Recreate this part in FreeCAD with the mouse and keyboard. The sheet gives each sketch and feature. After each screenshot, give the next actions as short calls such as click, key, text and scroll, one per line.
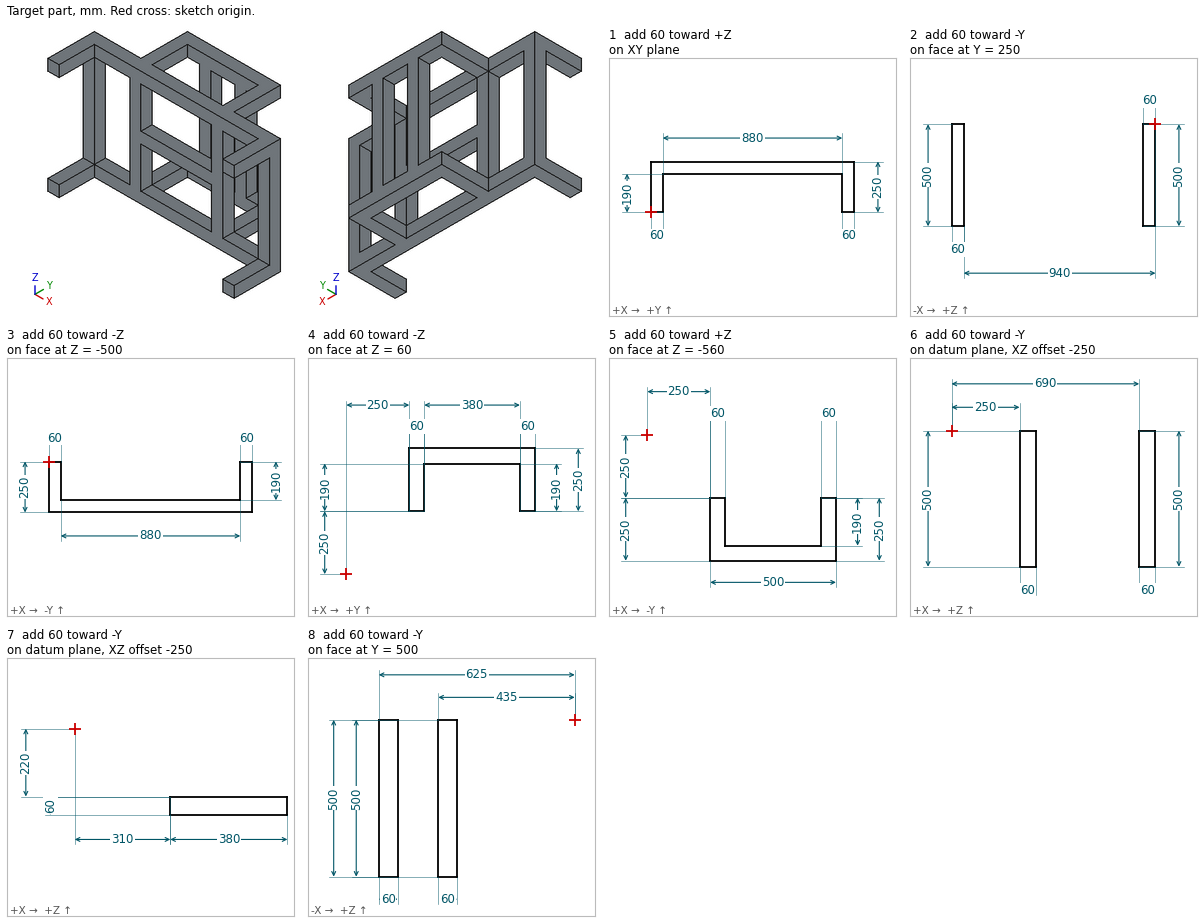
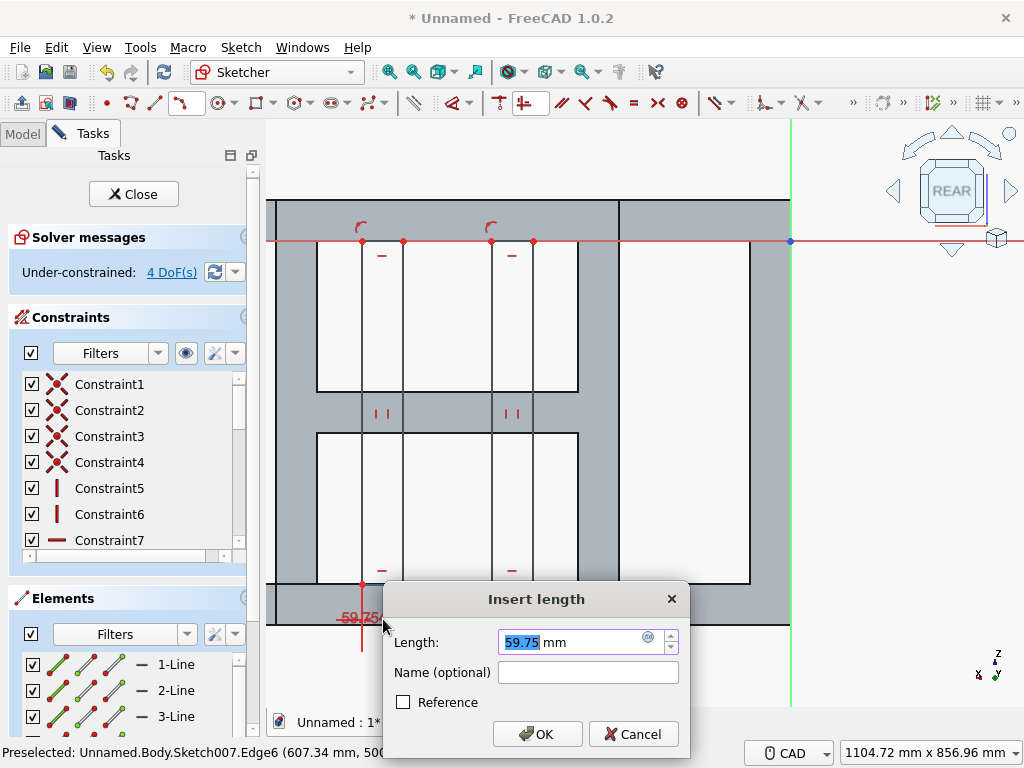
text(60)
key(Return)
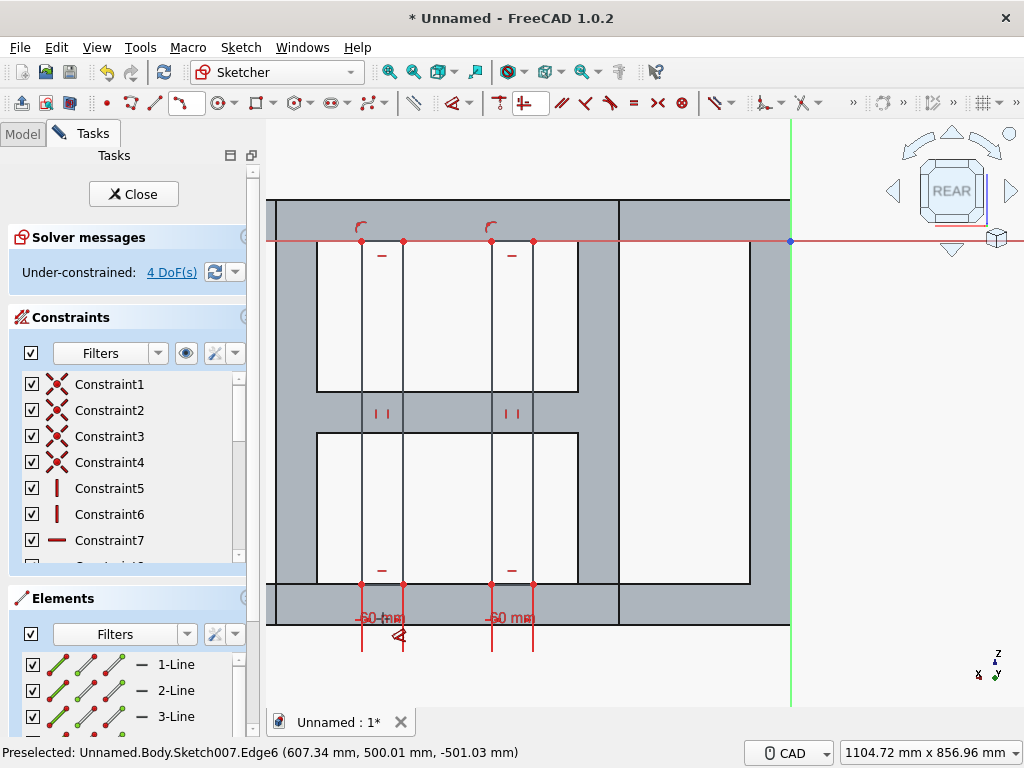
click(492, 344)
click(458, 413)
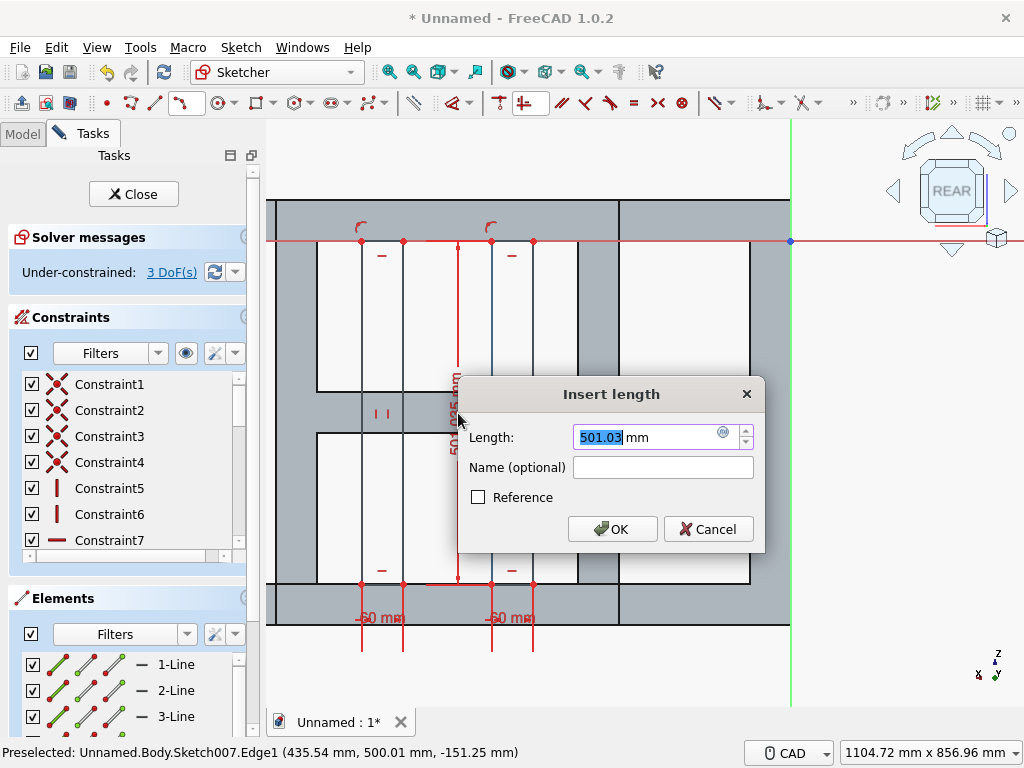
text(500)
key(Return)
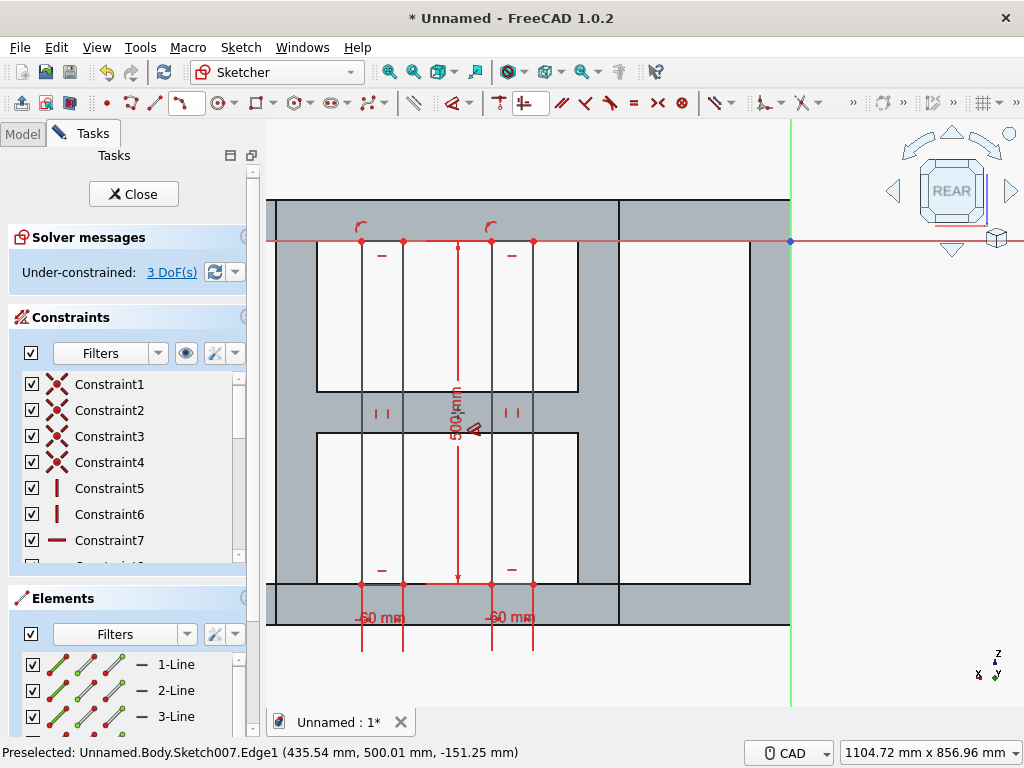
click(362, 344)
click(328, 413)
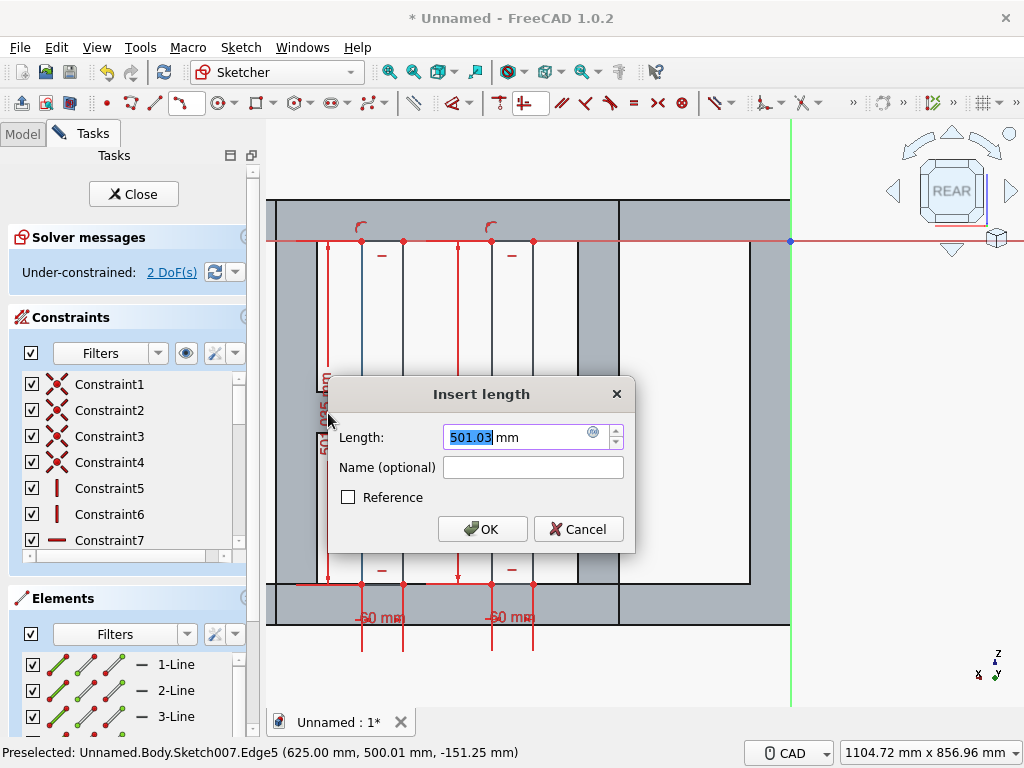
text(500)
key(Return)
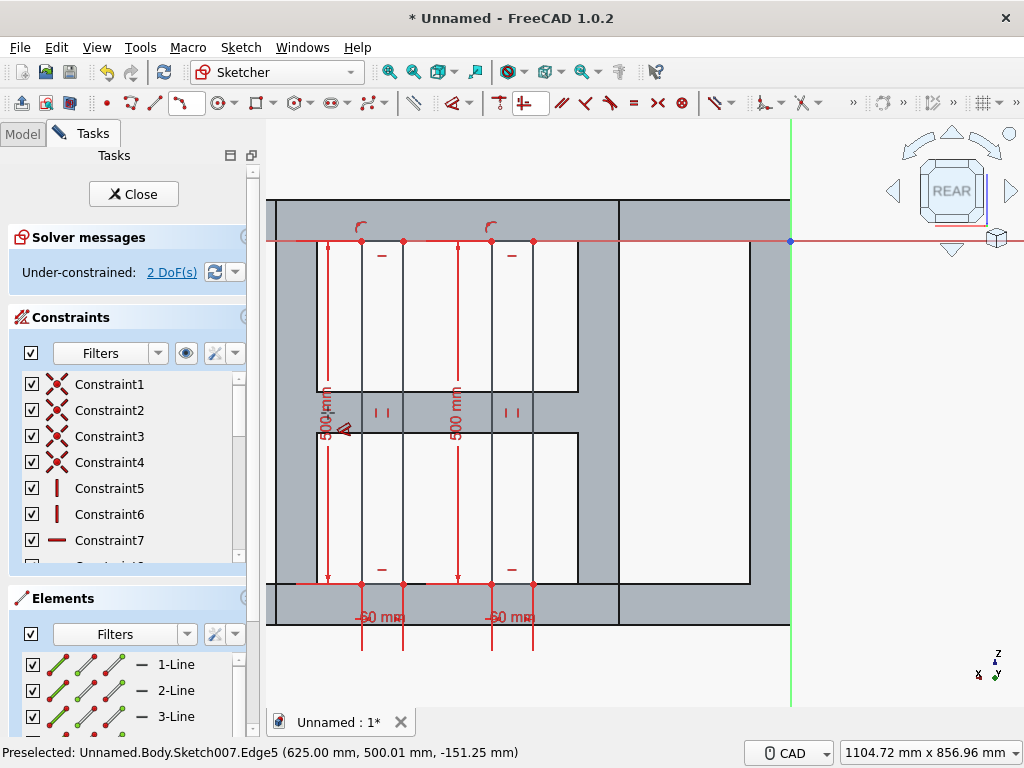
click(492, 241)
click(641, 207)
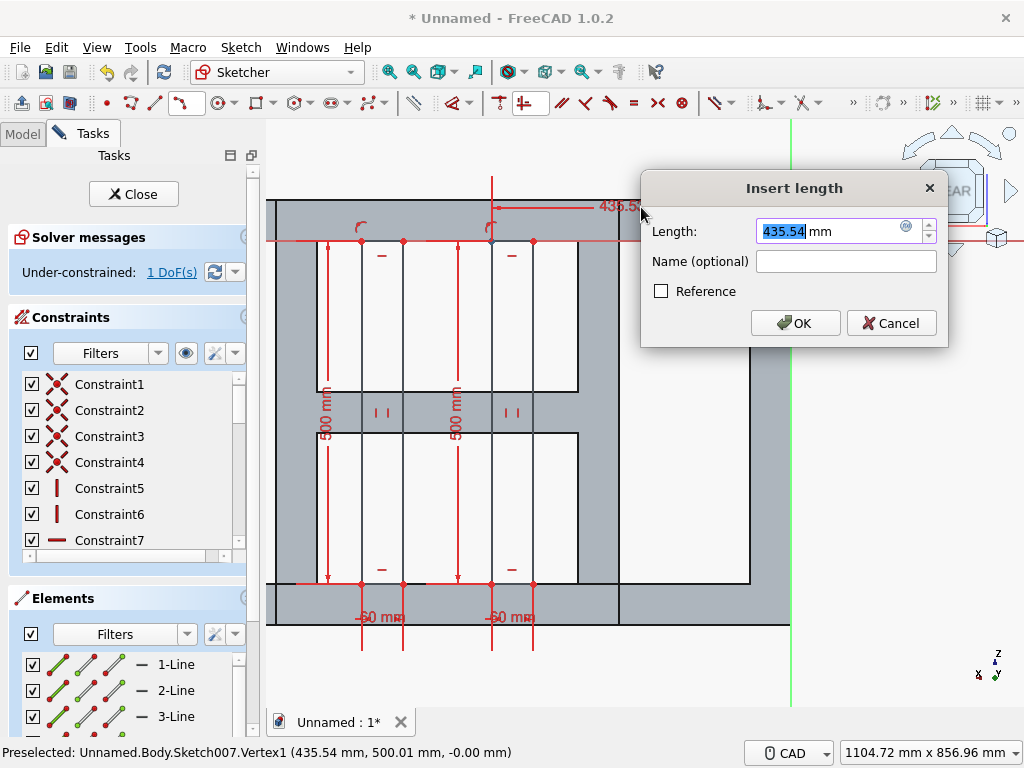
text(435)
key(Return)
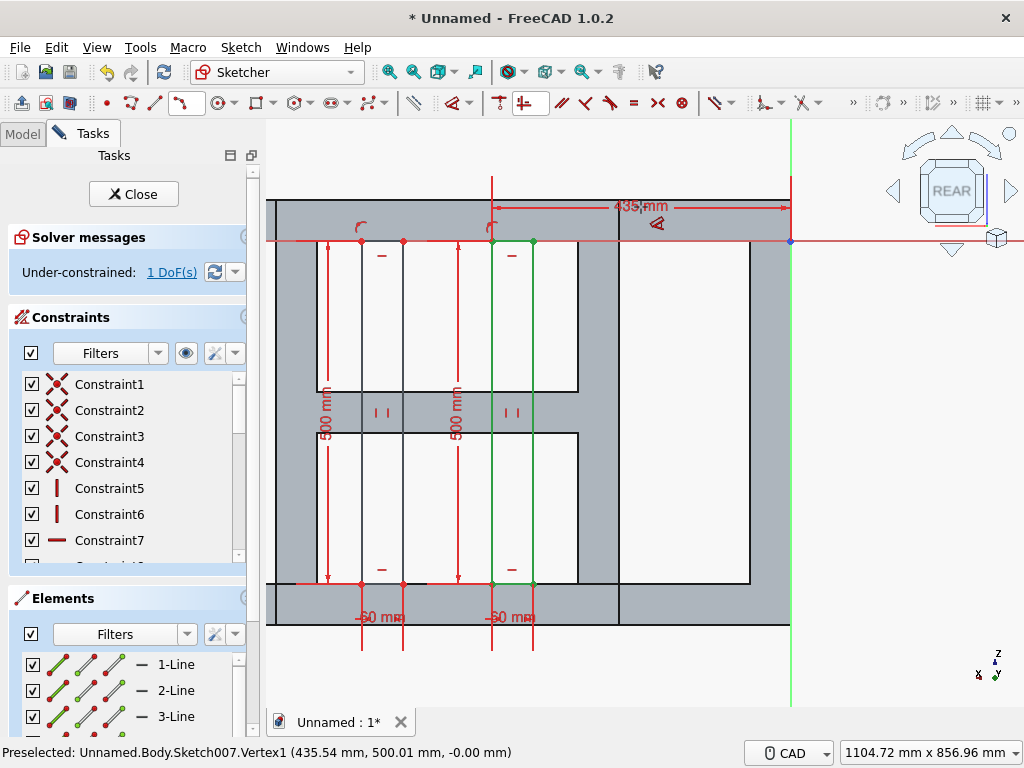
click(362, 241)
click(478, 207)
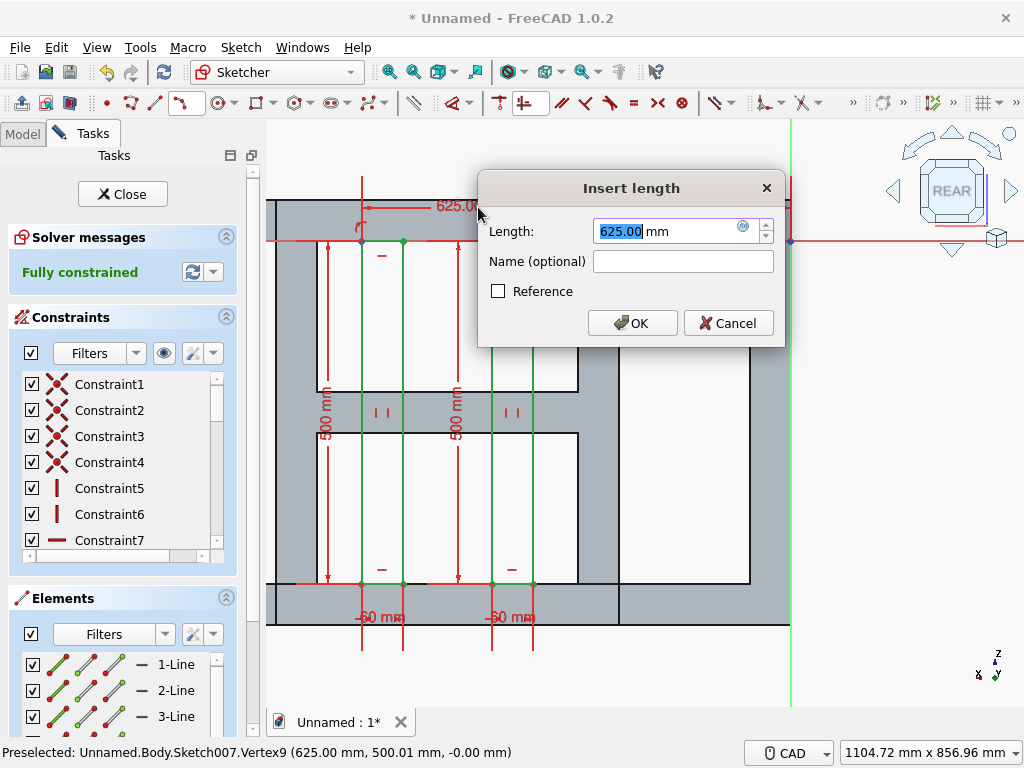
text(625)
key(Return)
key(Escape)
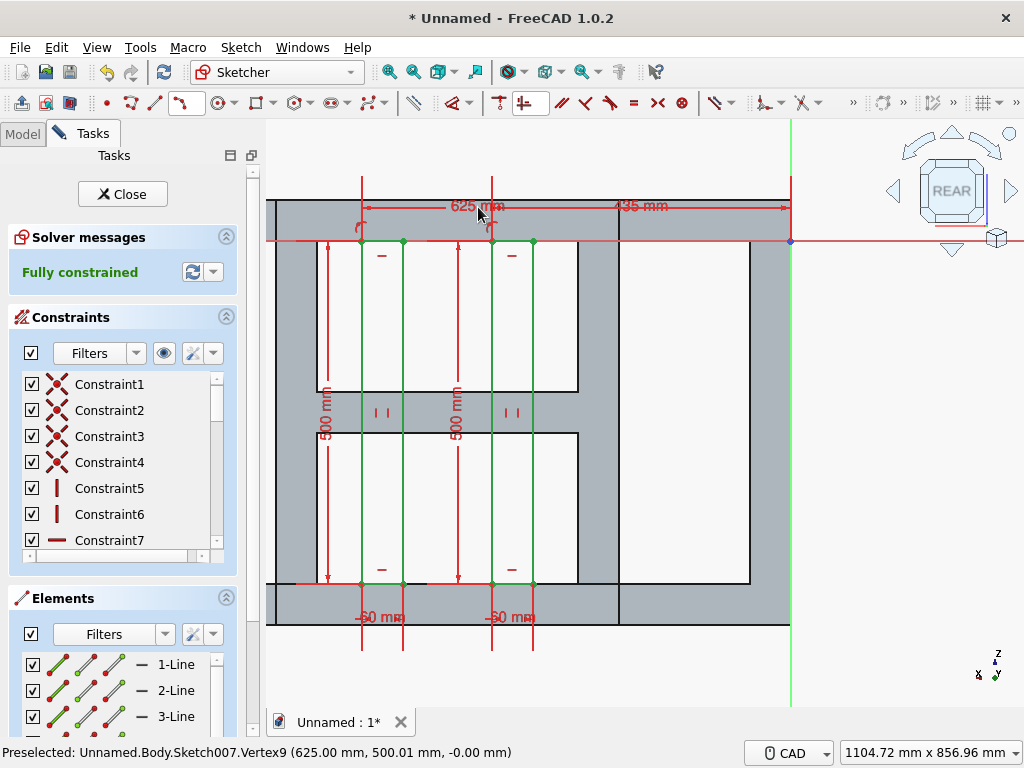
click(123, 194)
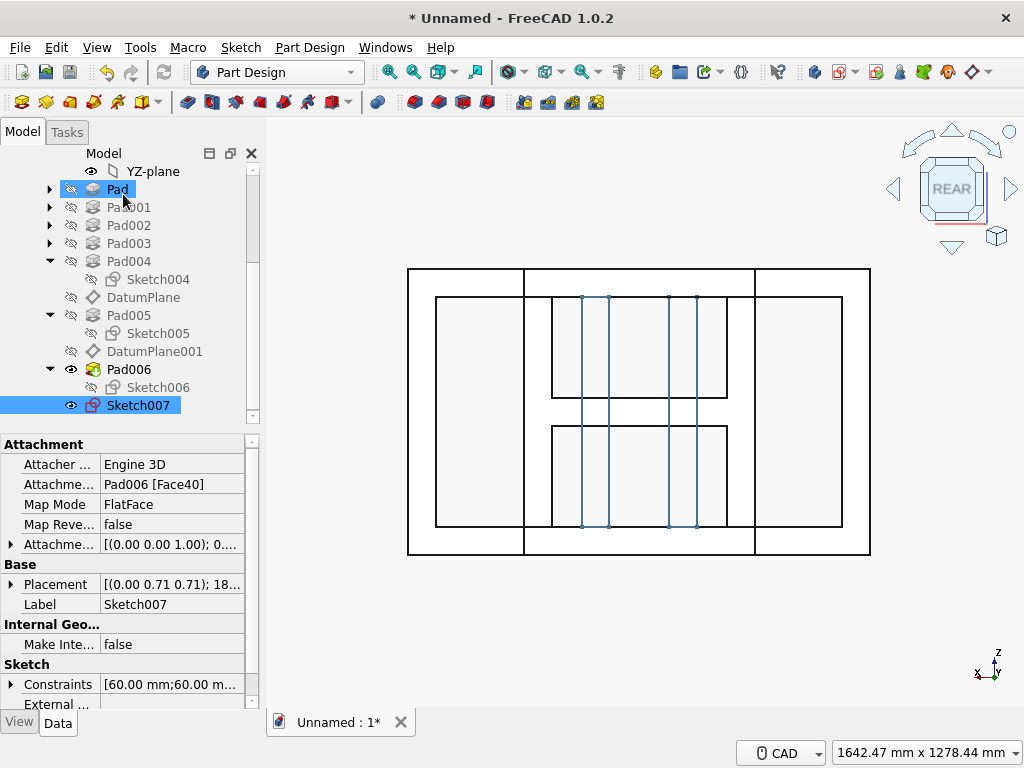
click(22, 102)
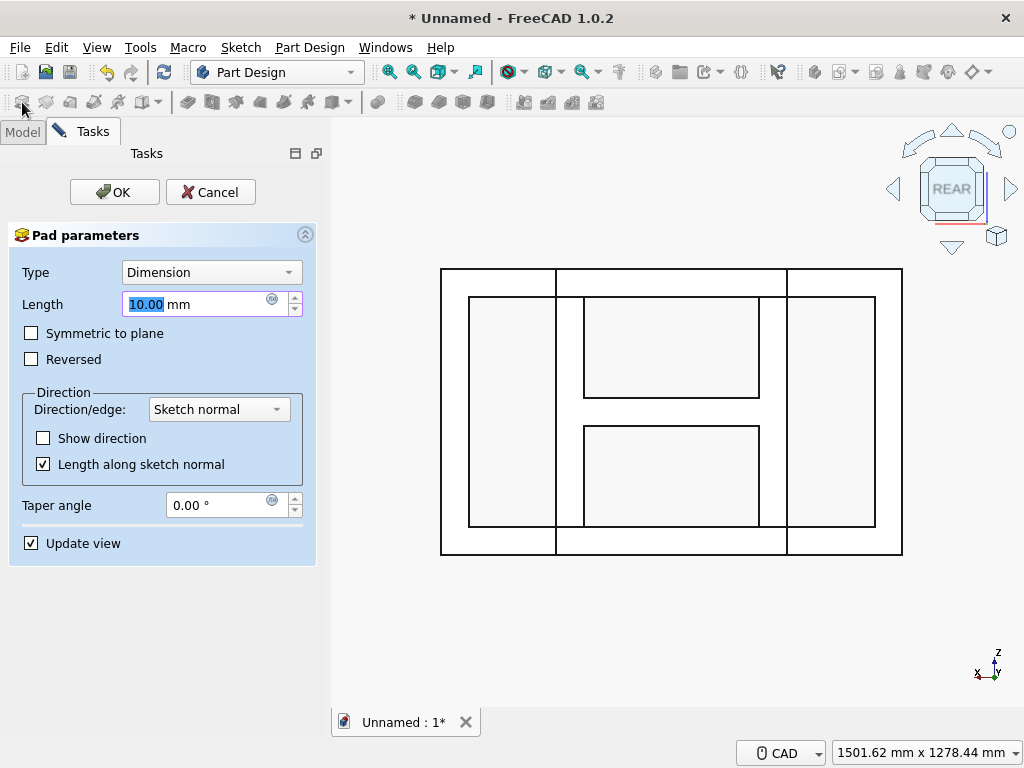
text(60)
key(Tab)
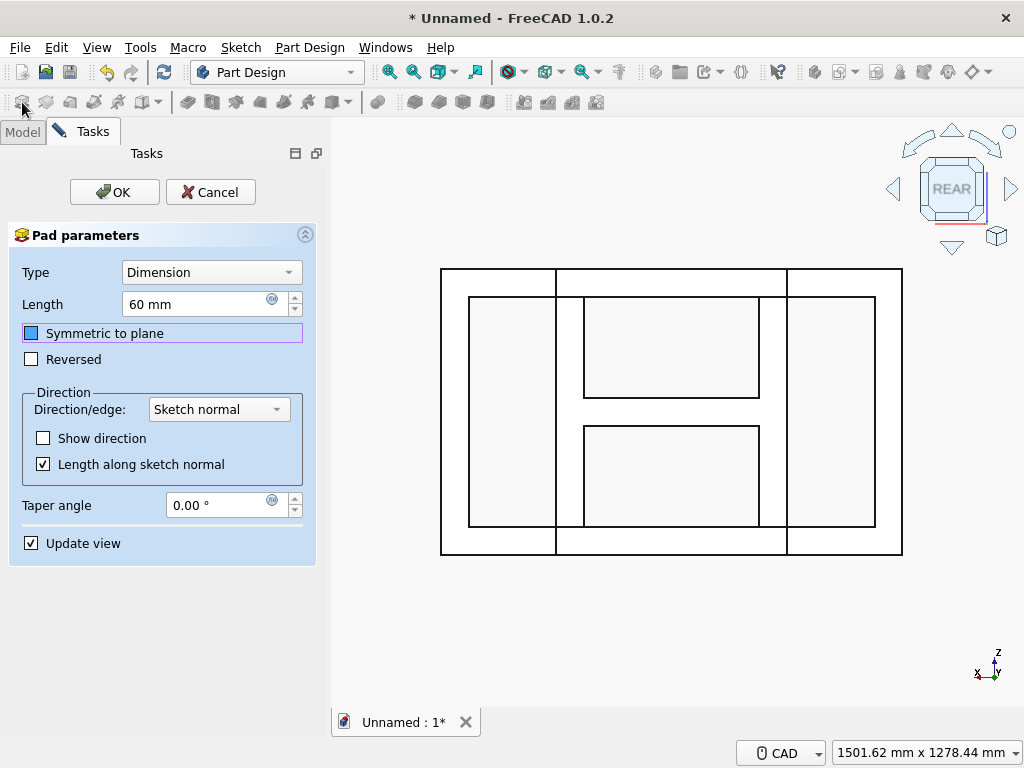
click(30, 359)